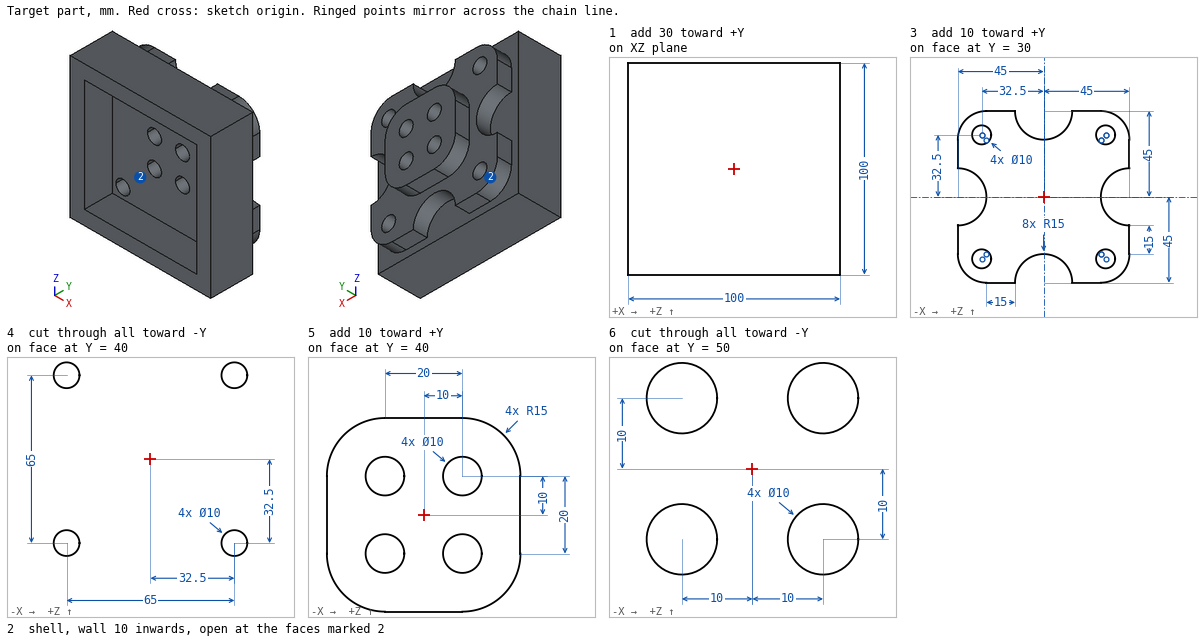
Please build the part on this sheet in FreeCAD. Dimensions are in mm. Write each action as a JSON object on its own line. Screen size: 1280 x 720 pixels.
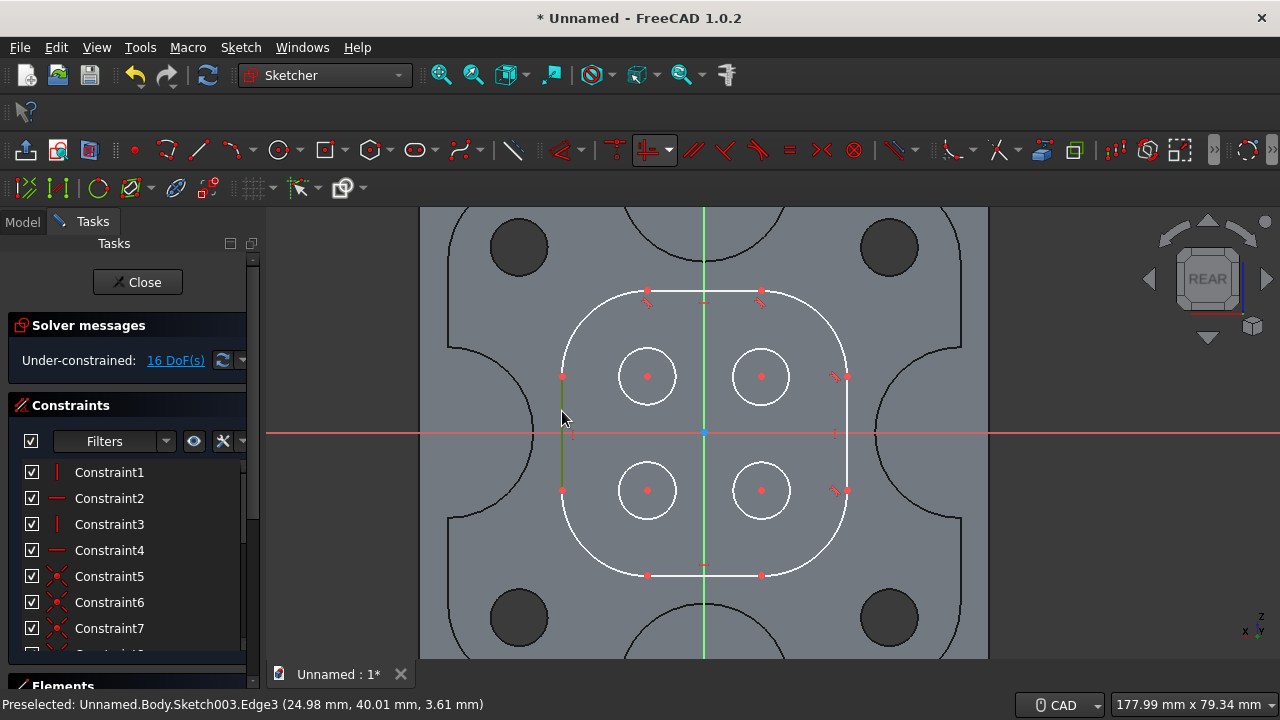
{"action": "left_click", "coordinate": [608, 300]}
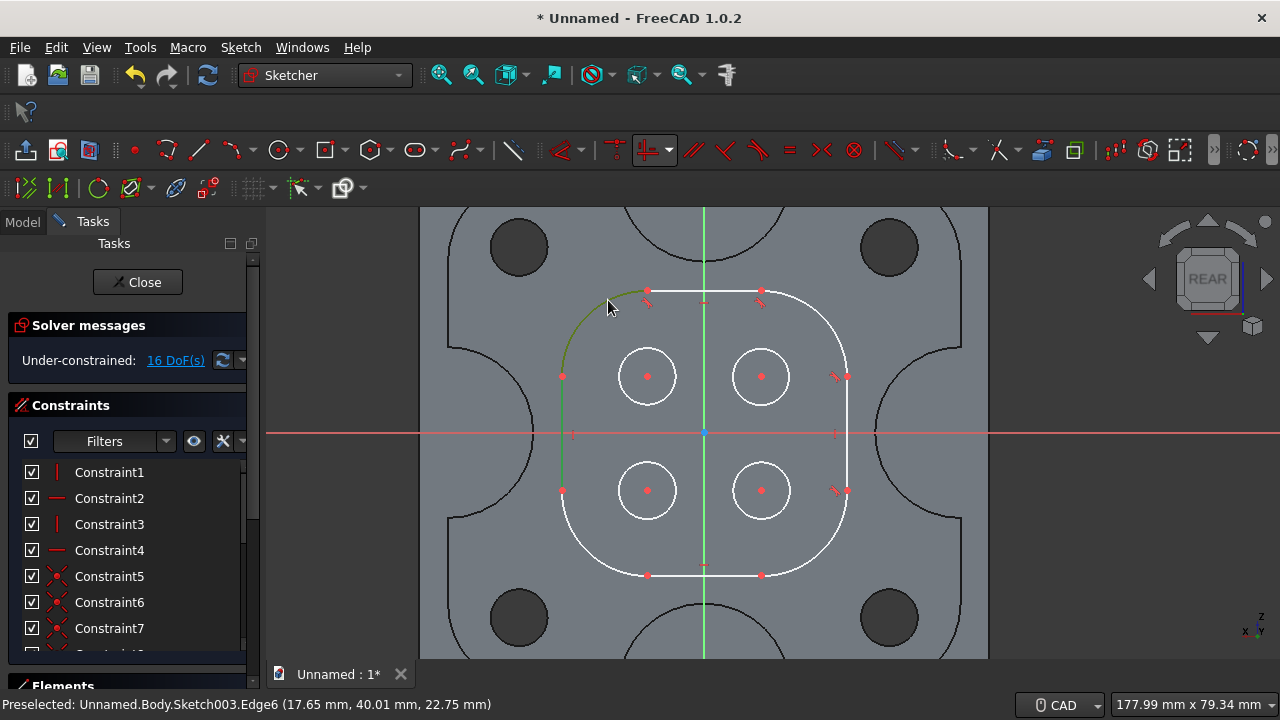
{"action": "left_click", "coordinate": [758, 150]}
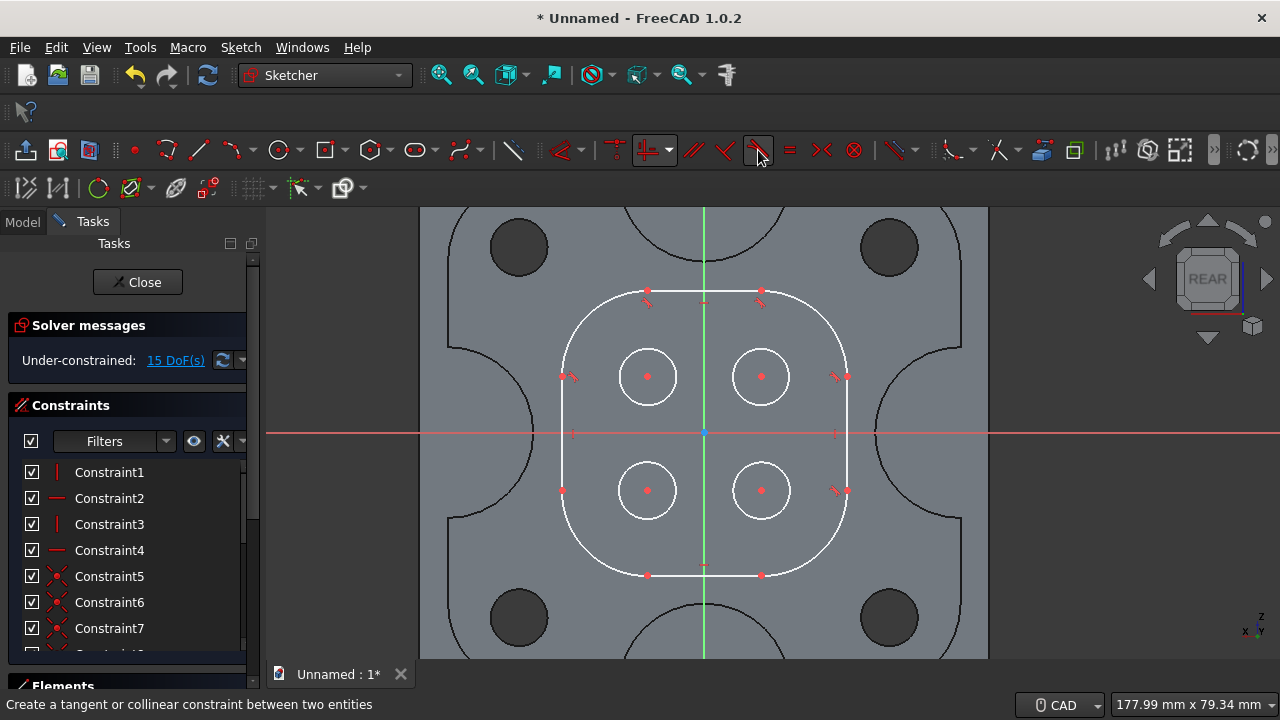
{"action": "left_click", "coordinate": [562, 411]}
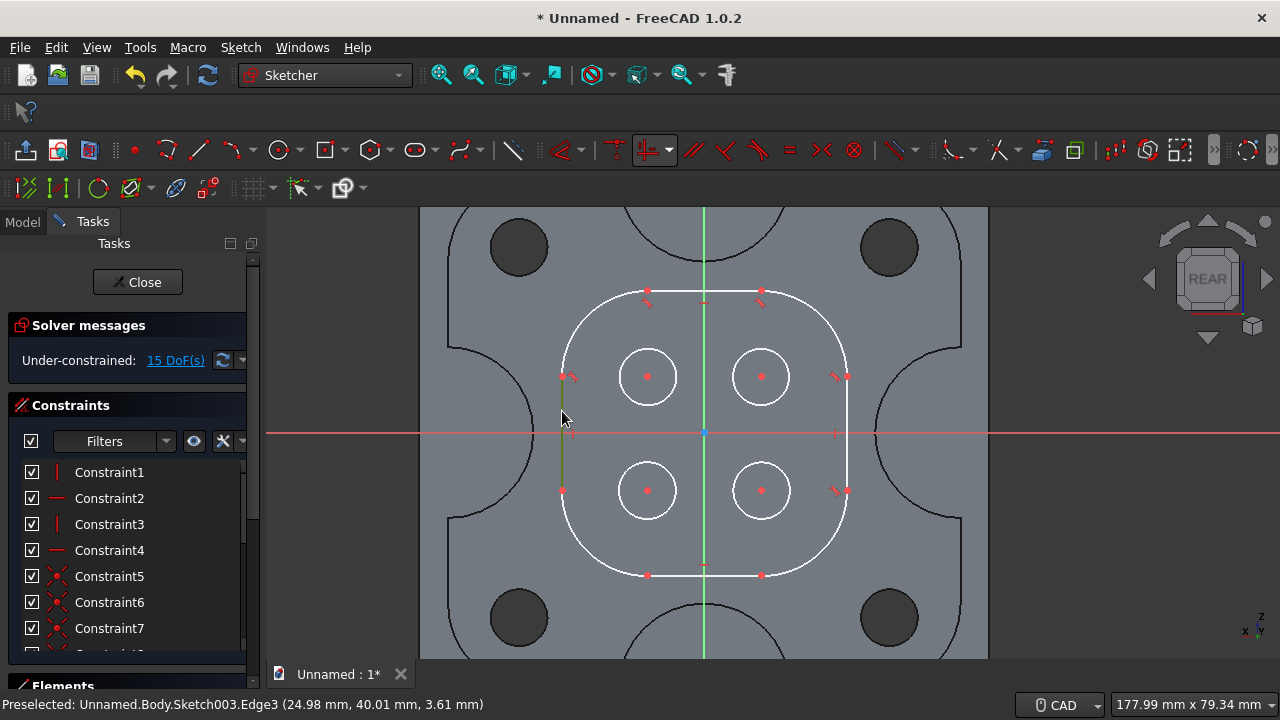
{"action": "left_click", "coordinate": [571, 530]}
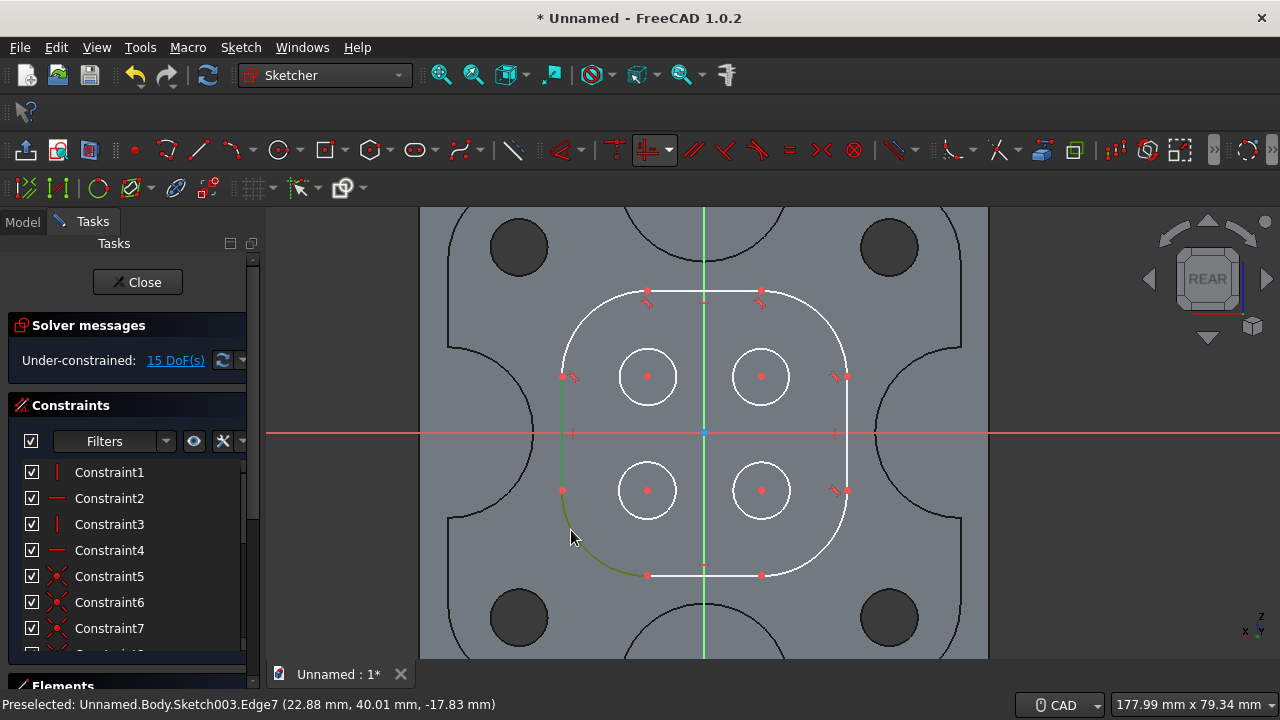
{"action": "left_click", "coordinate": [758, 150]}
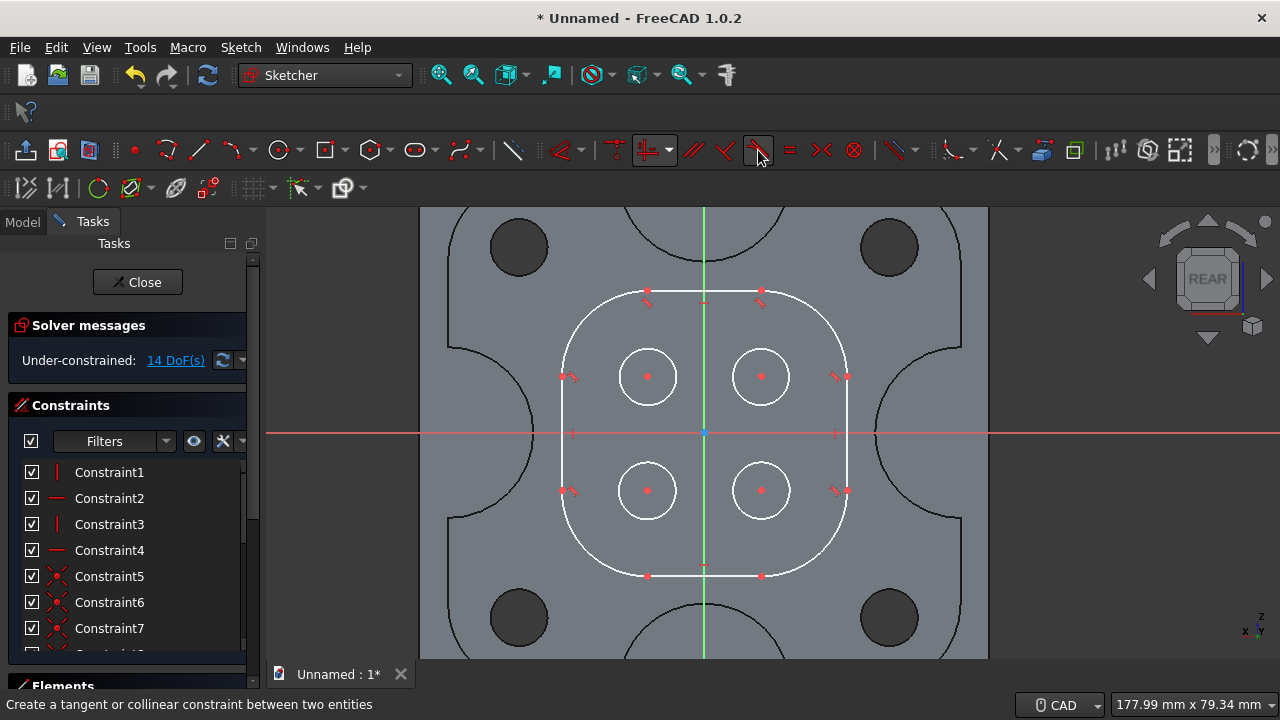
{"action": "left_click", "coordinate": [681, 576]}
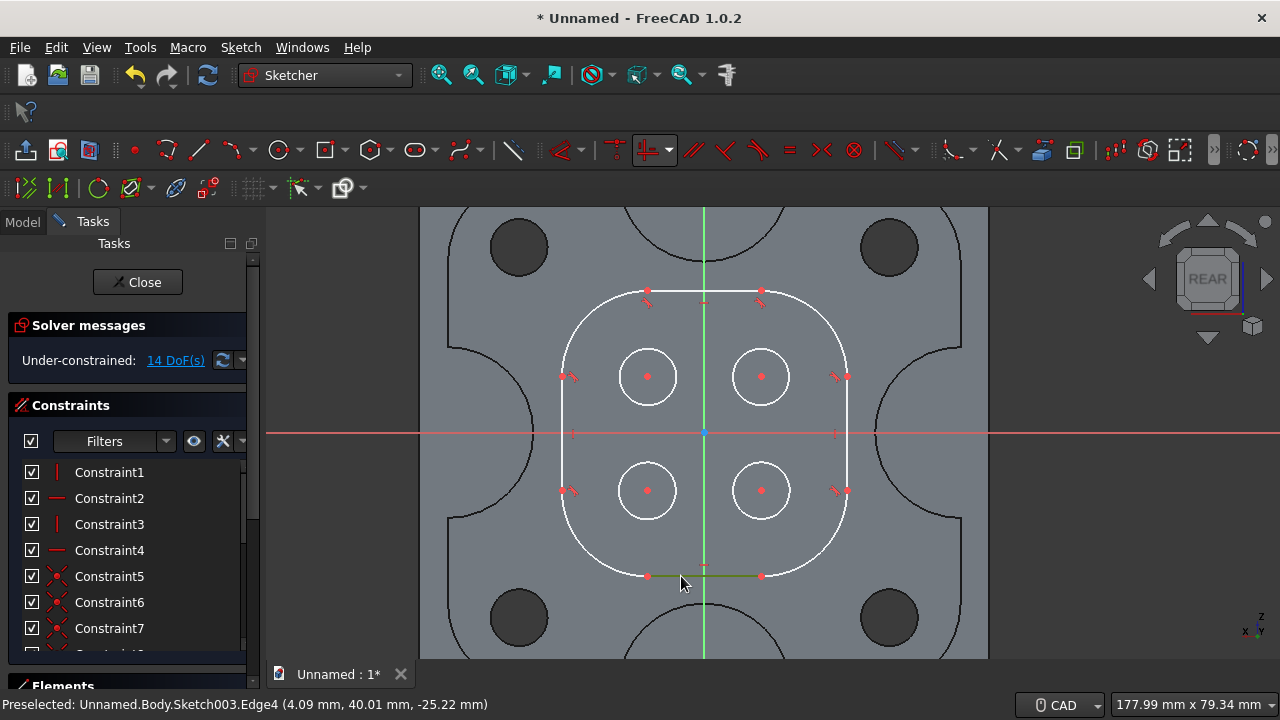
{"action": "left_click", "coordinate": [571, 530]}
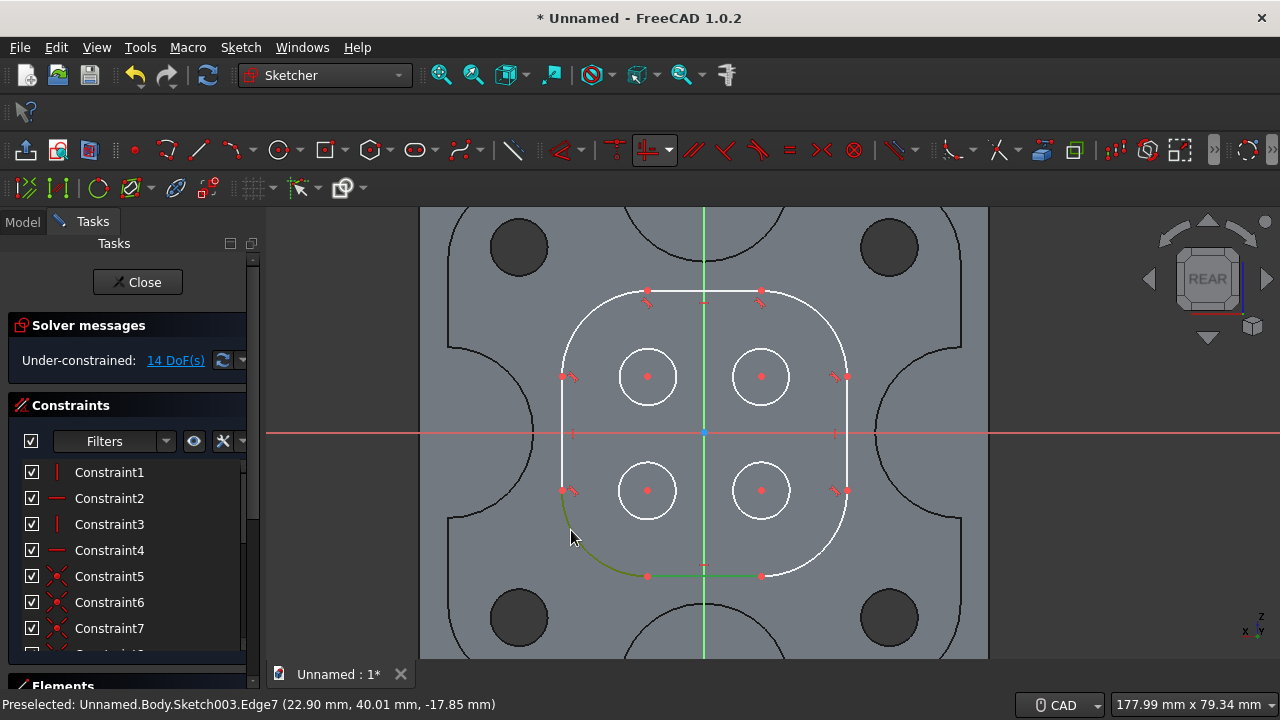
{"action": "left_click", "coordinate": [758, 150]}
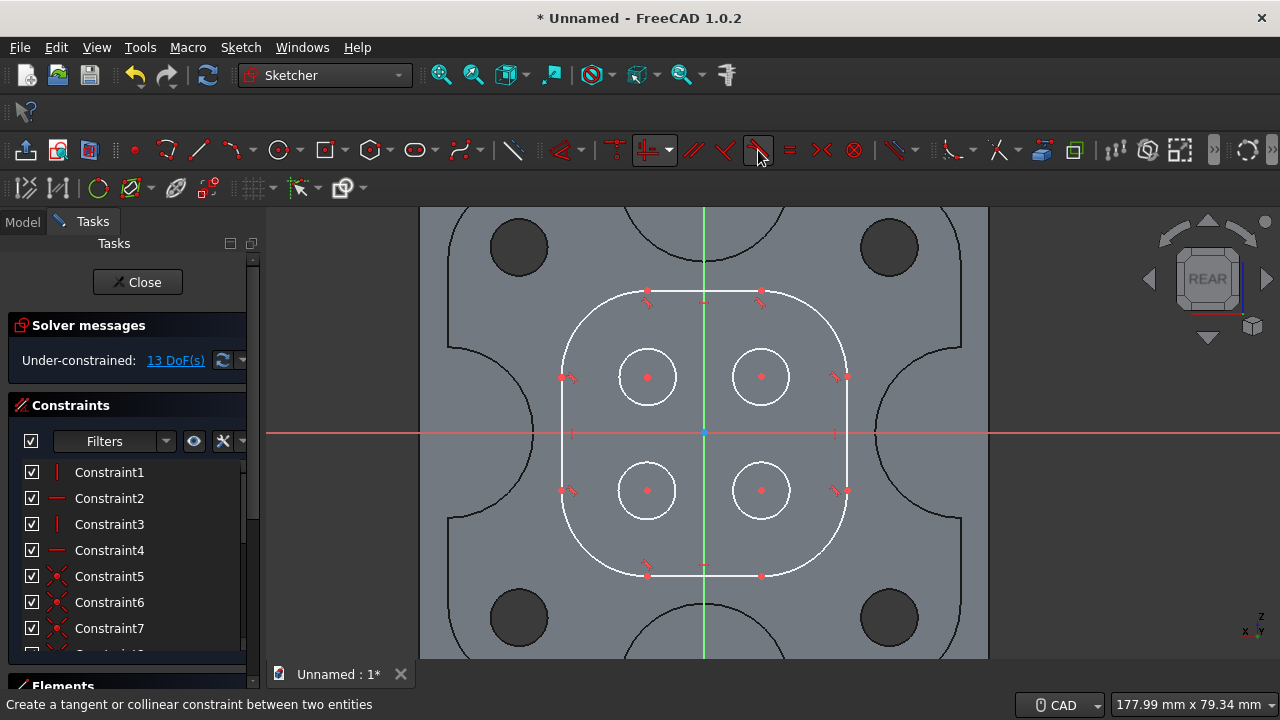
{"action": "left_click", "coordinate": [681, 576]}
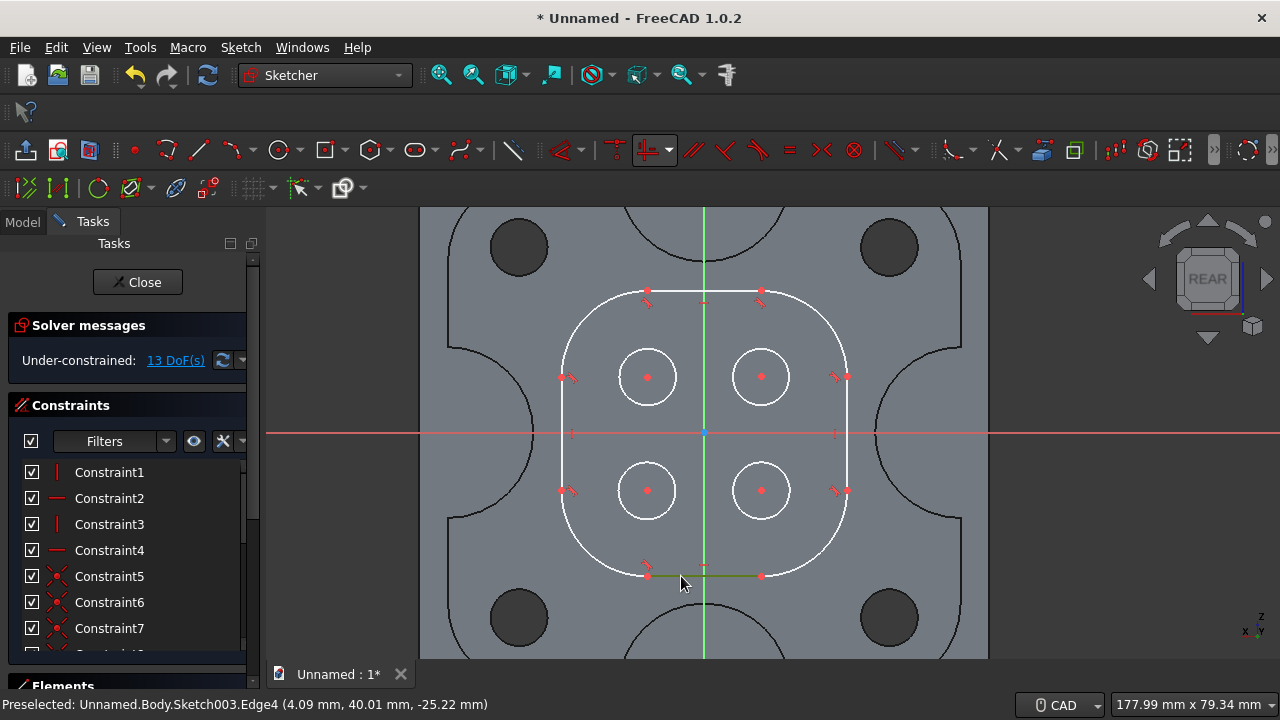
{"action": "left_click", "coordinate": [800, 567]}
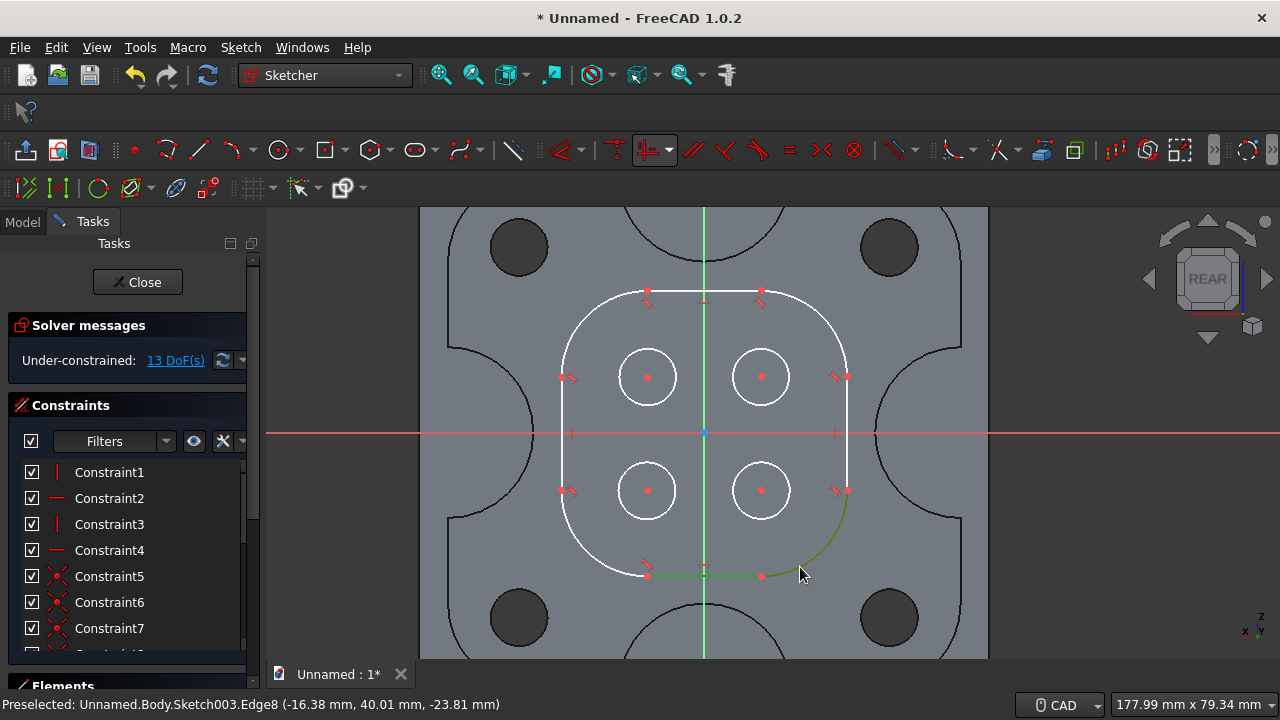
{"action": "left_click", "coordinate": [758, 150]}